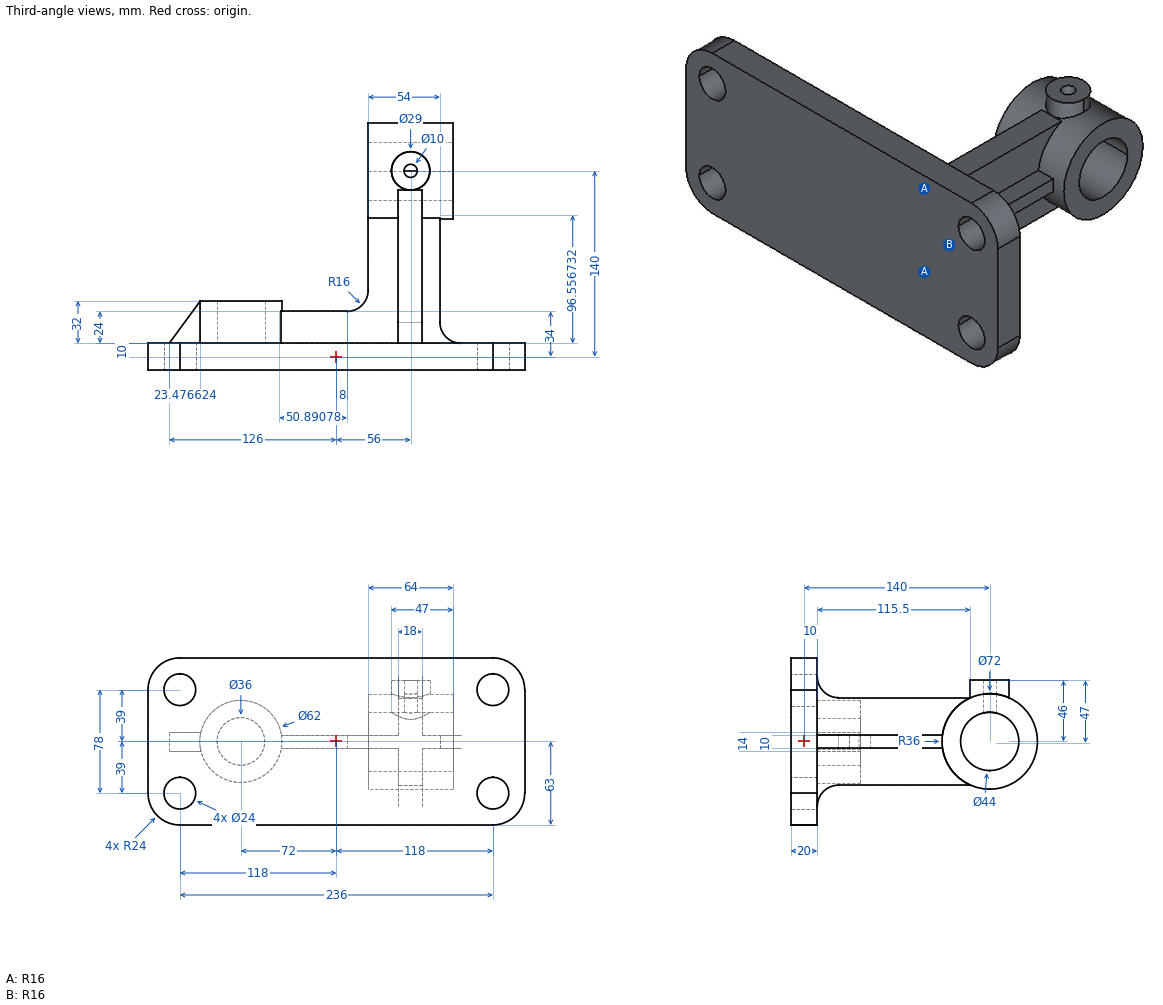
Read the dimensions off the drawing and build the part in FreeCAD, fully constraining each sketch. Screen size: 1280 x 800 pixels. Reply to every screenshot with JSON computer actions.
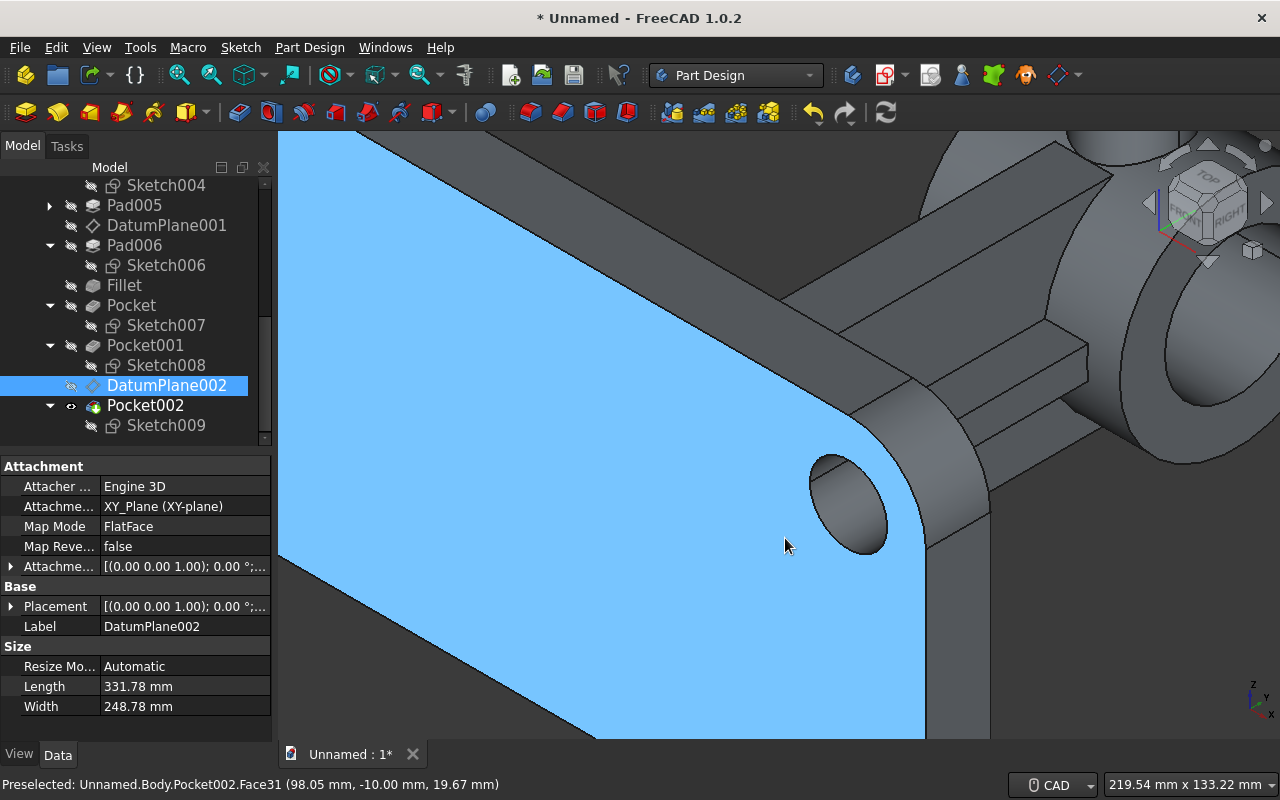
{"action": "left_click", "coordinate": [180, 76]}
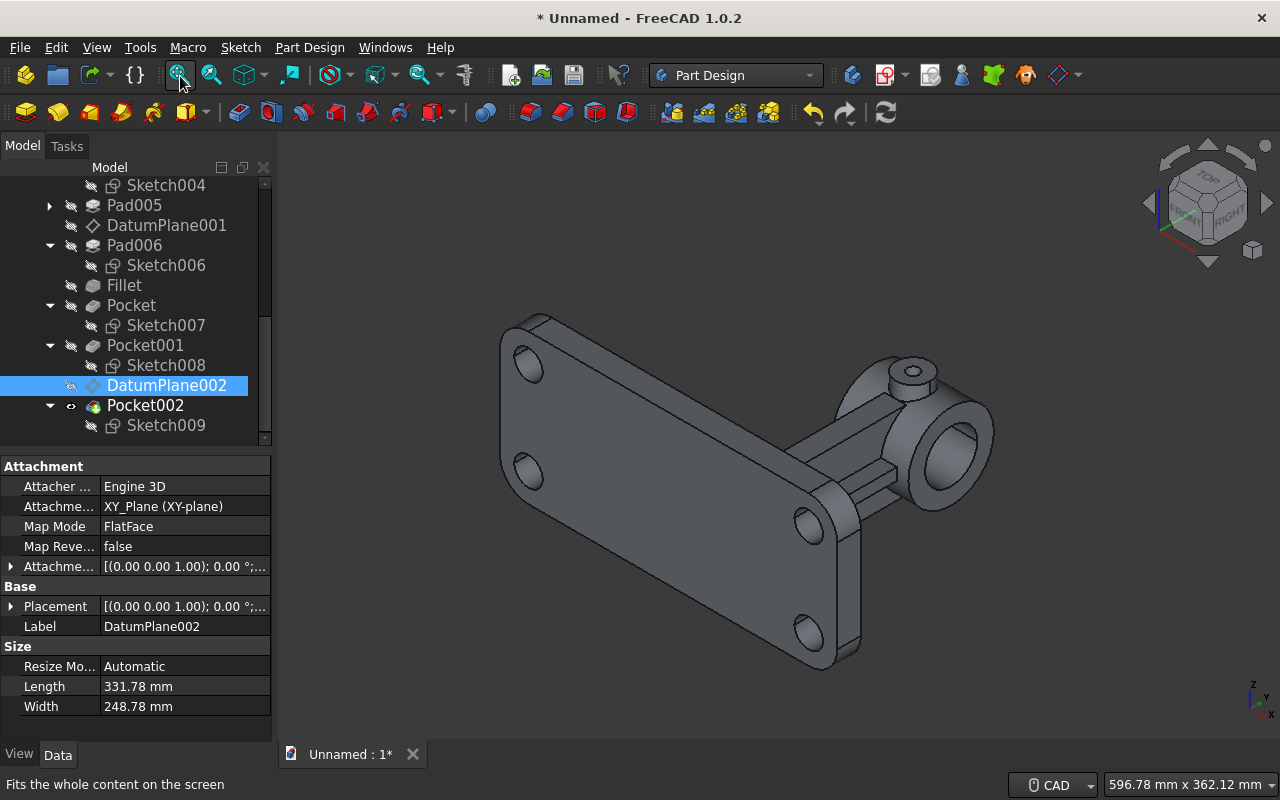
{"action": "key", "text": "1"}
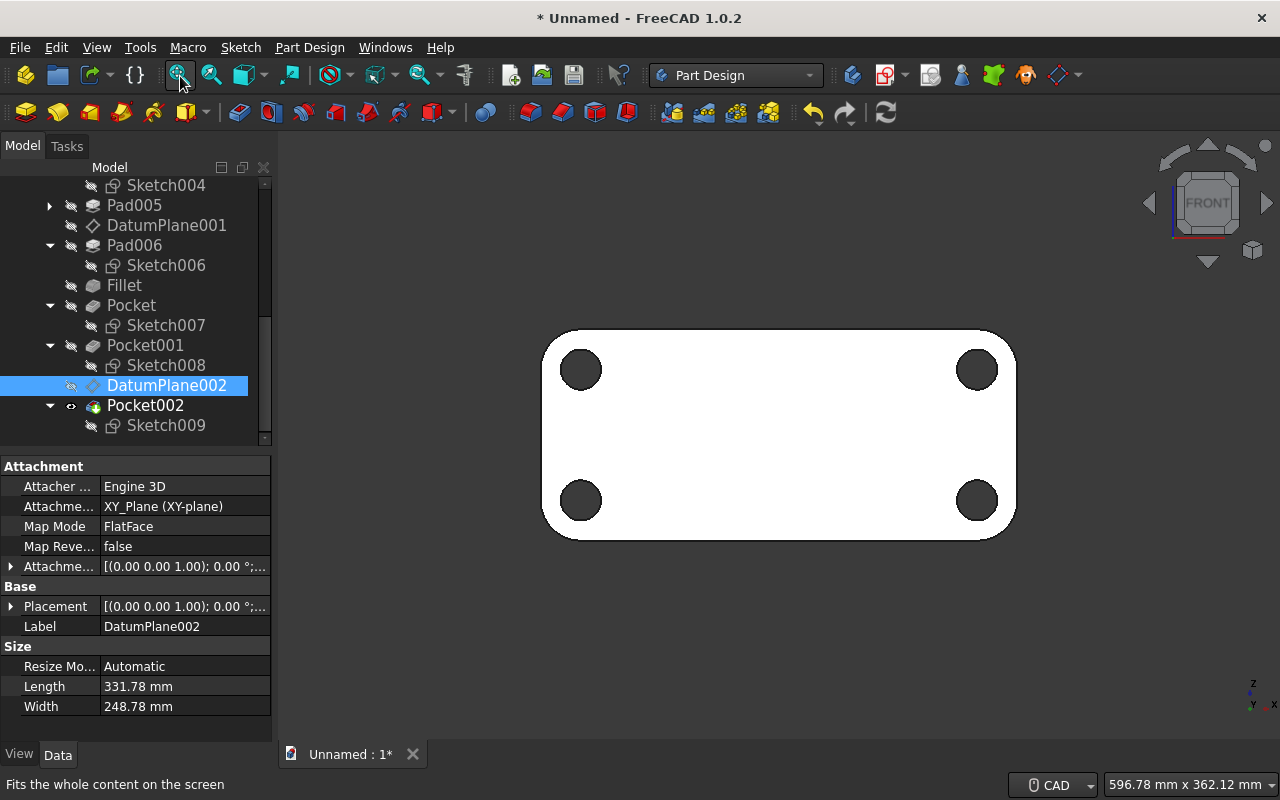
{"action": "scroll", "coordinate": [910, 434], "scroll_direction": "up", "scroll_amount": 5}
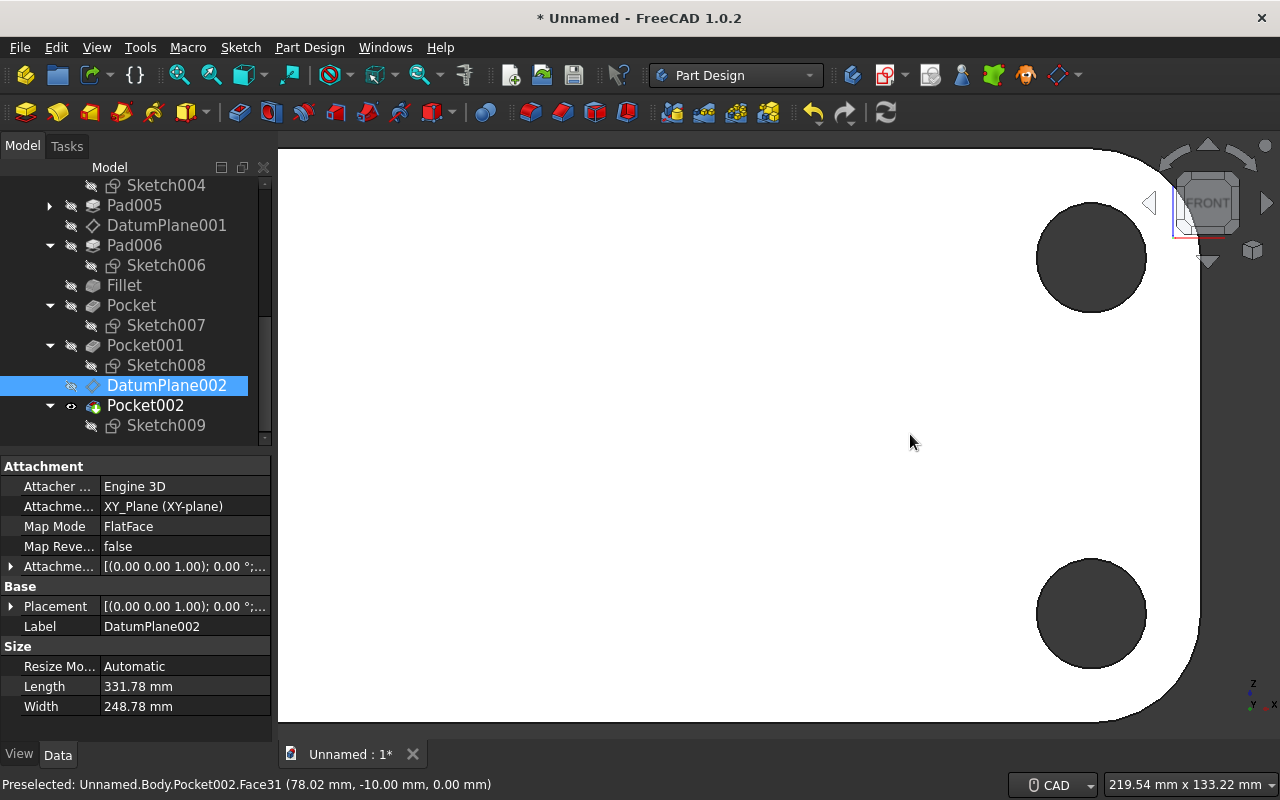
{"action": "left_click", "coordinate": [180, 76]}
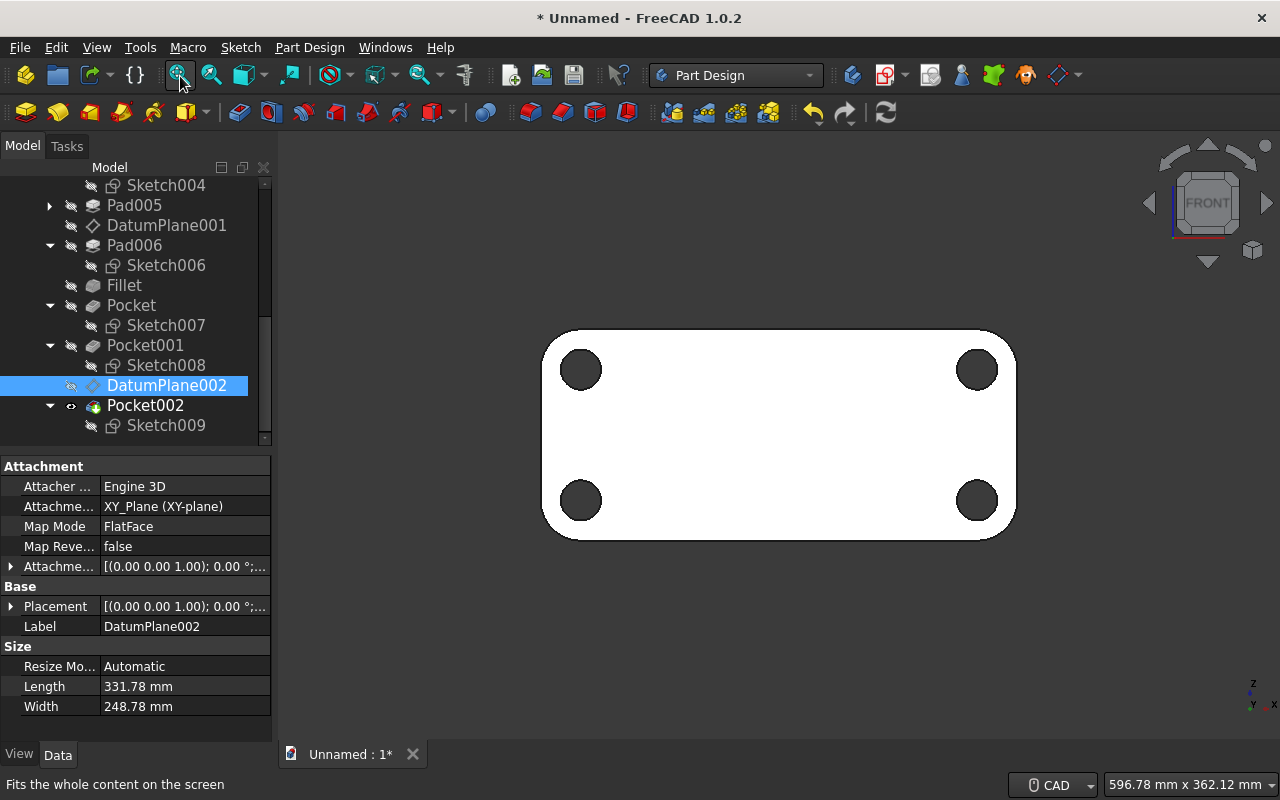
{"action": "key", "text": "3"}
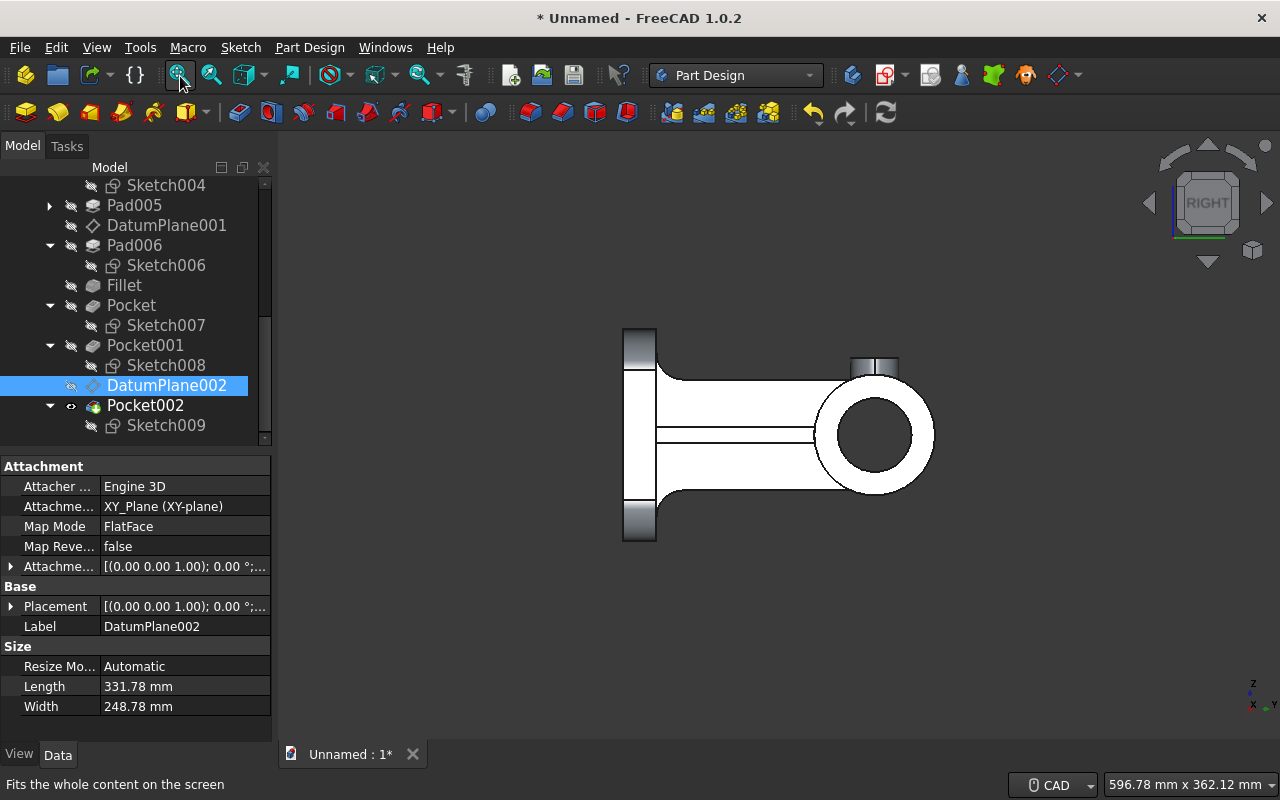
{"action": "left_click", "coordinate": [180, 76]}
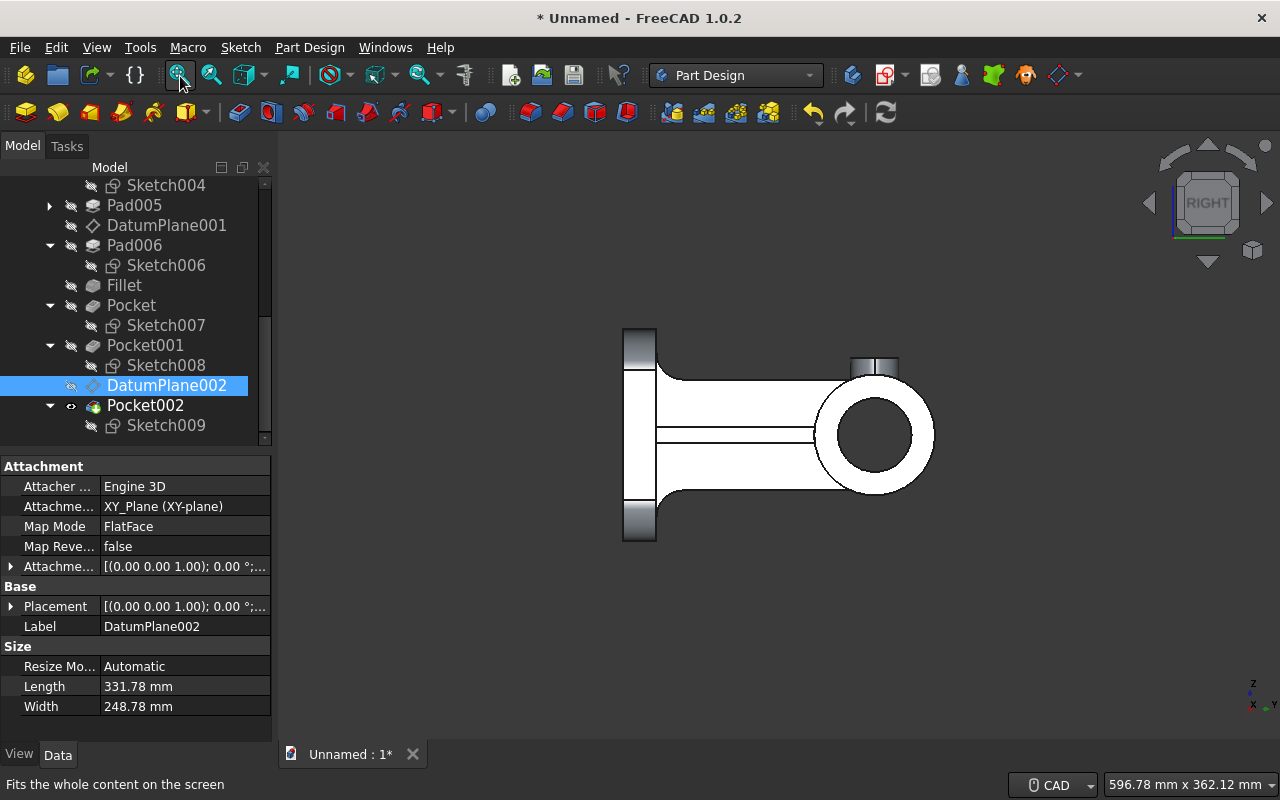
{"action": "scroll", "coordinate": [656, 434], "scroll_direction": "up", "scroll_amount": 5}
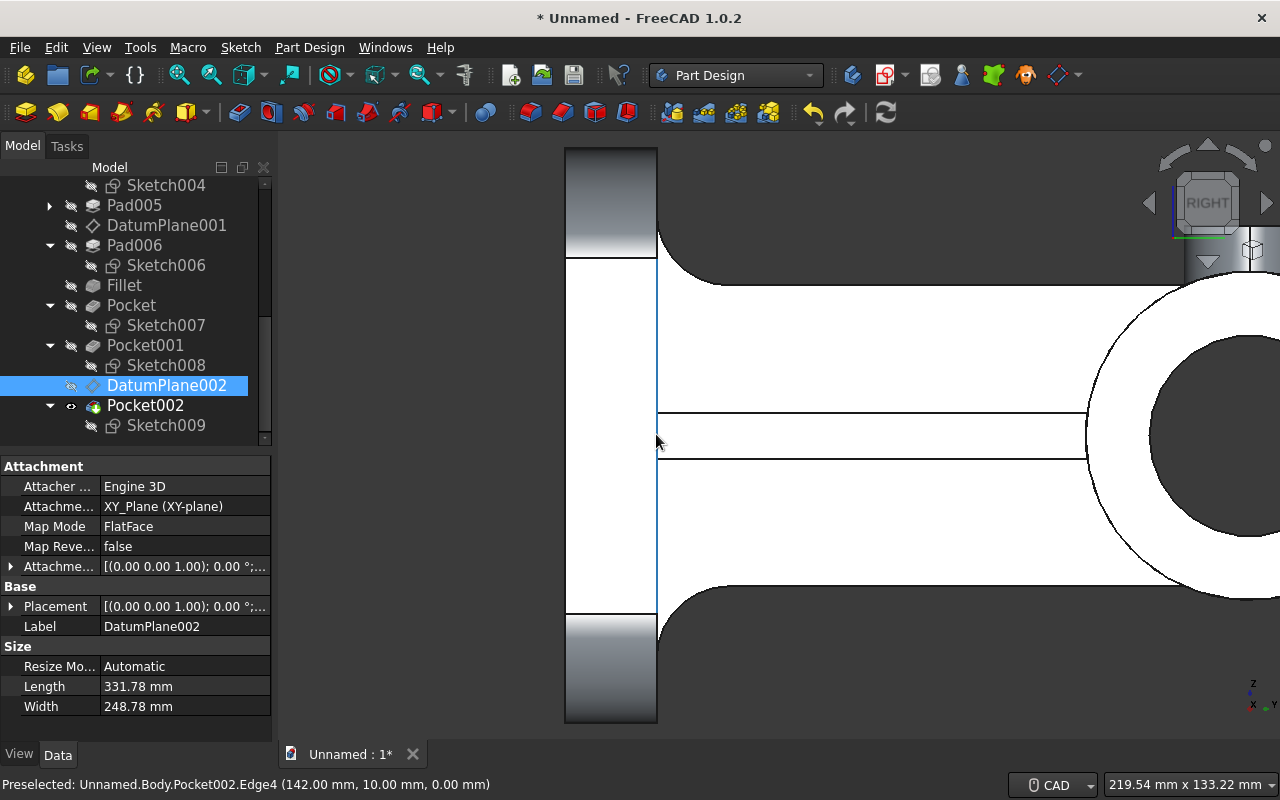
{"action": "left_click", "coordinate": [180, 76]}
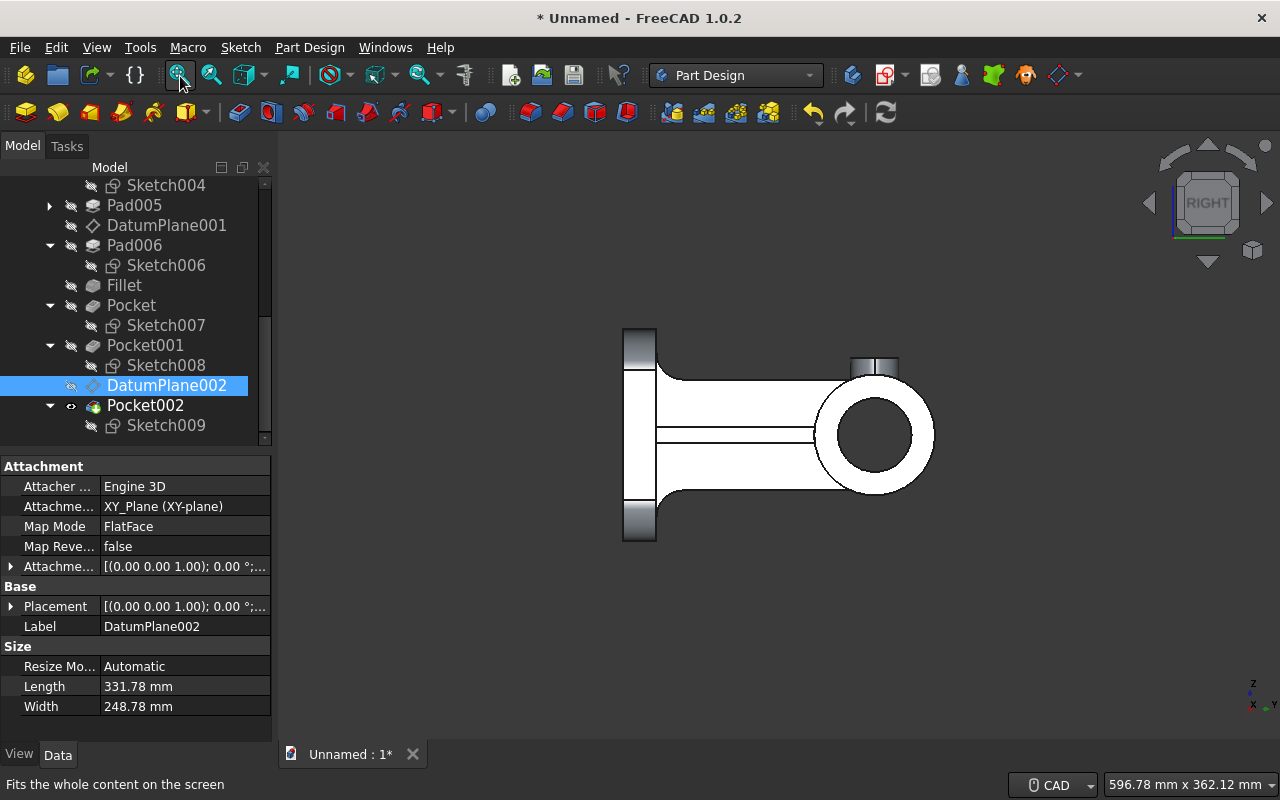
{"action": "key", "text": "5"}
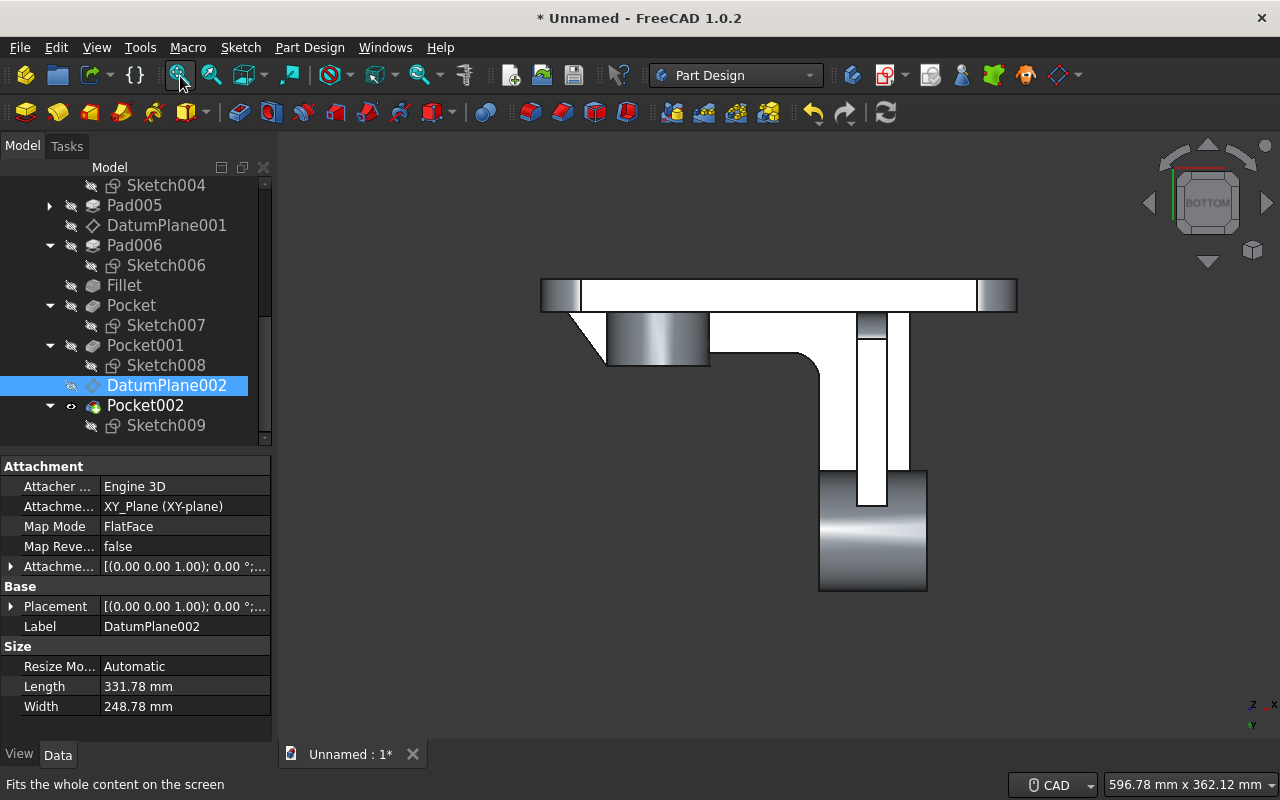
{"action": "scroll", "coordinate": [910, 311], "scroll_direction": "up", "scroll_amount": 5}